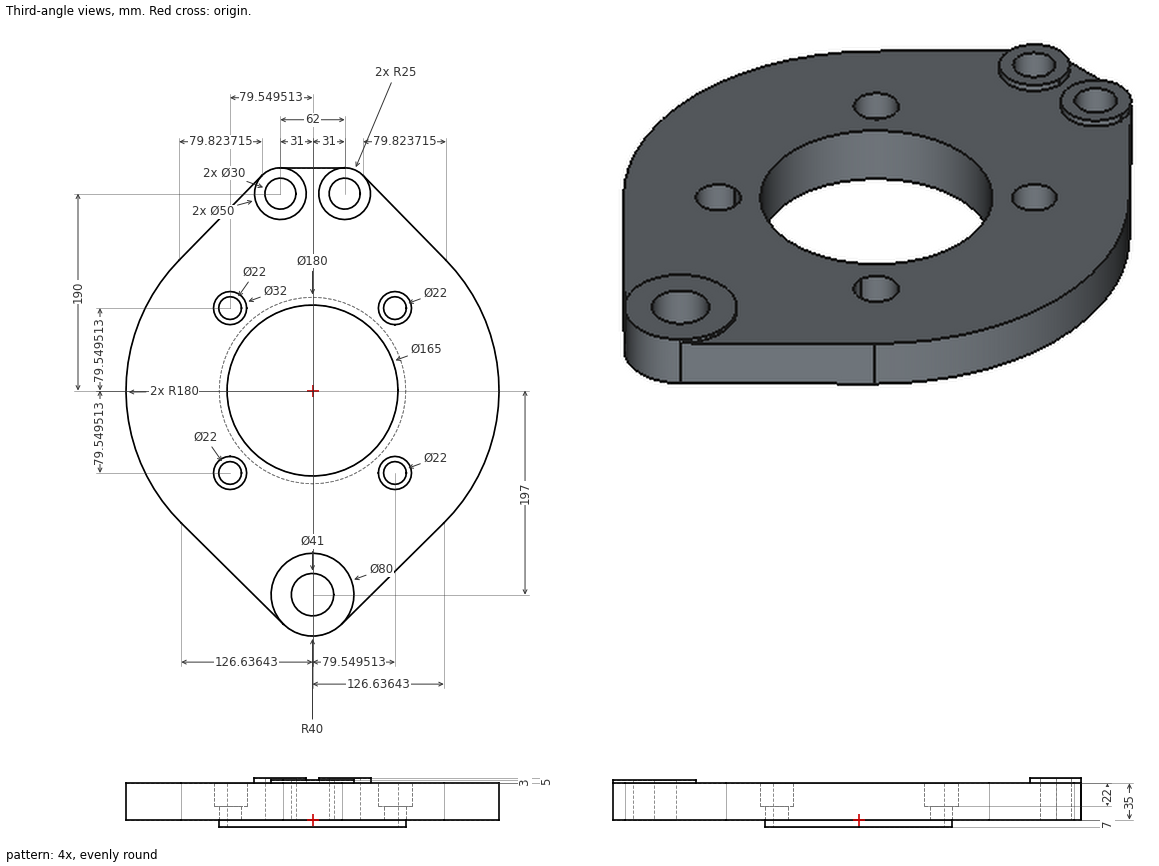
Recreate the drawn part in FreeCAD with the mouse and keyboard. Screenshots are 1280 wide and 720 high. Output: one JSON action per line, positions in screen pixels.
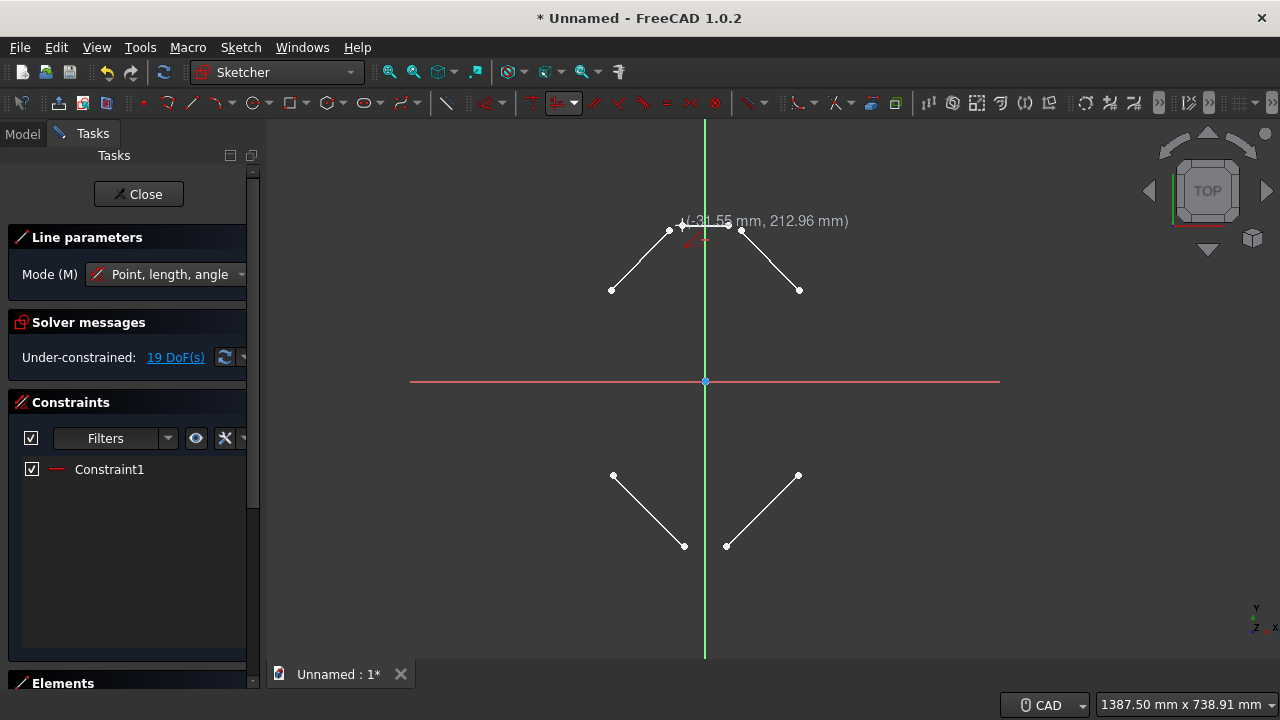
{"action": "key", "text": "g 3 a"}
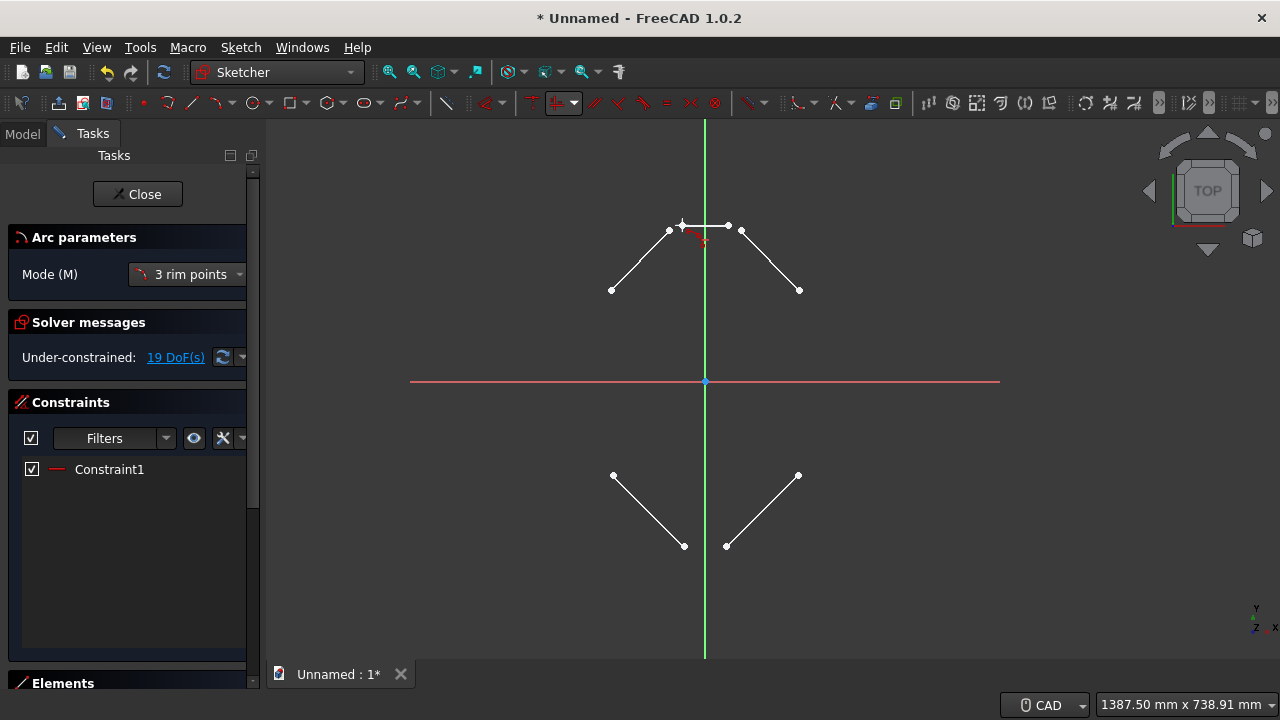
{"action": "left_click", "coordinate": [611, 291]}
{"action": "left_click", "coordinate": [613, 476]}
{"action": "left_click", "coordinate": [575, 362]}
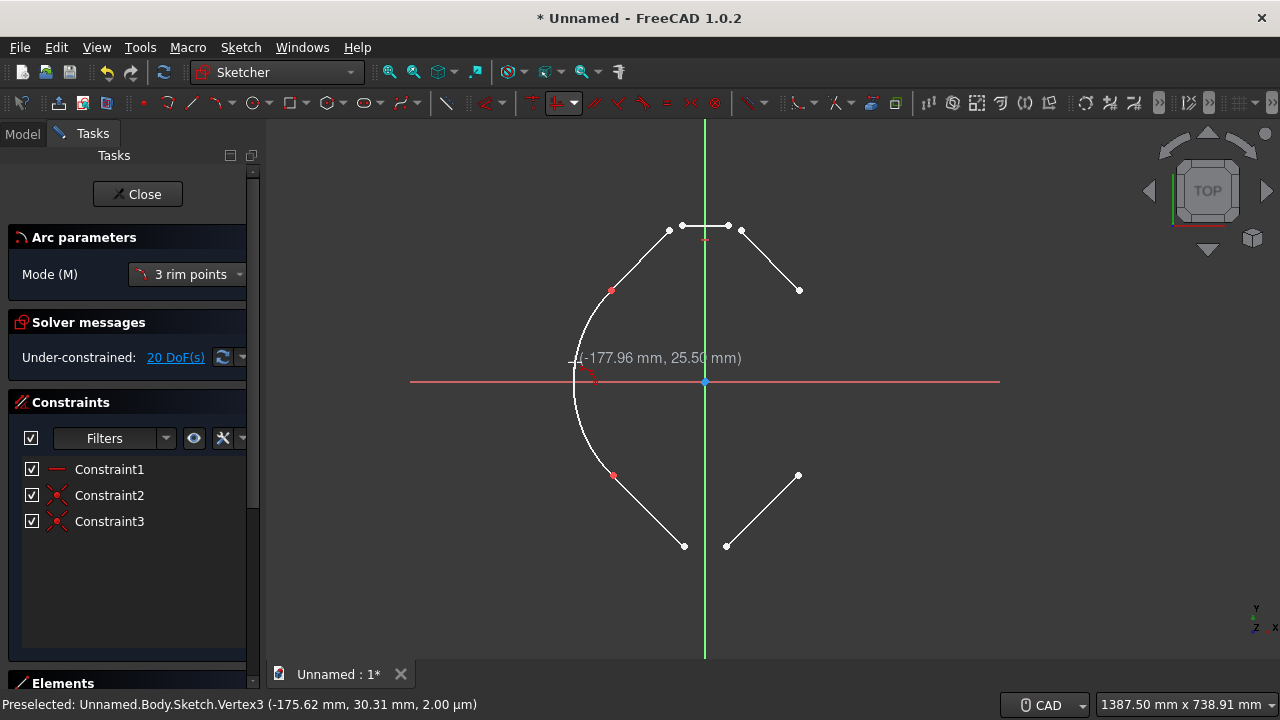
{"action": "left_click", "coordinate": [684, 547]}
{"action": "left_click", "coordinate": [726, 547]}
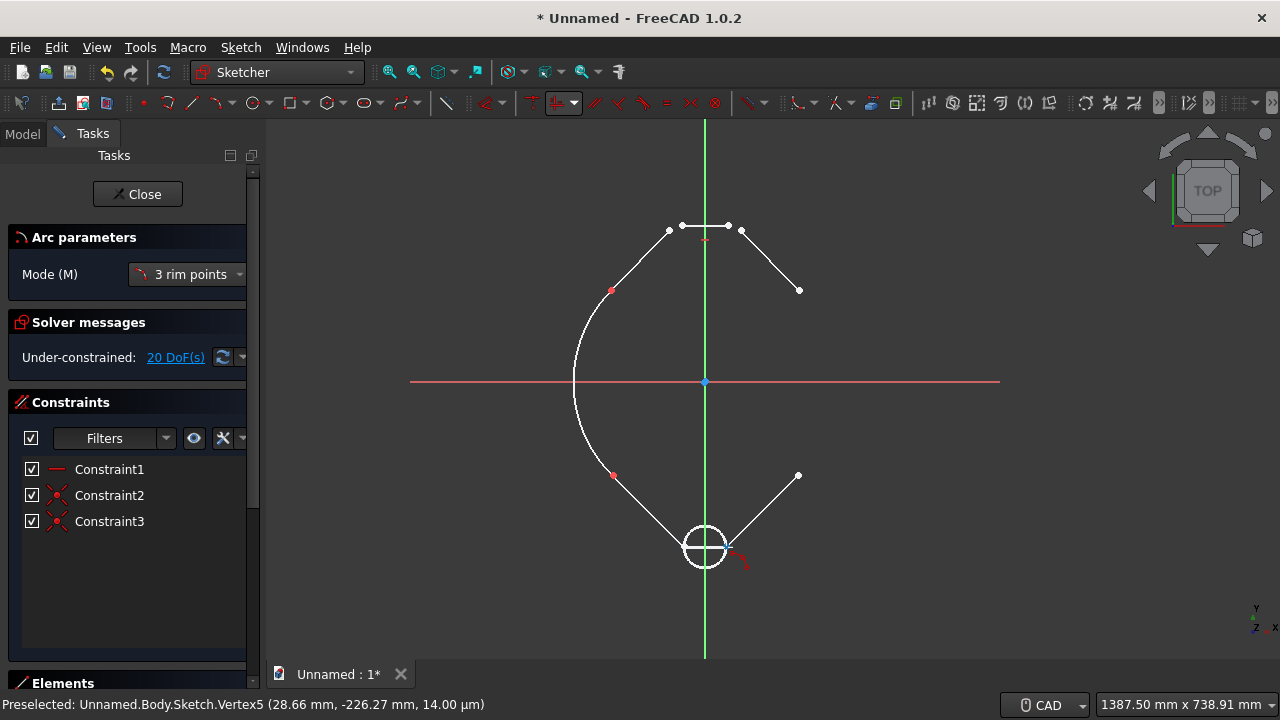
{"action": "scroll", "coordinate": [696, 553], "scroll_direction": "up", "scroll_amount": 5}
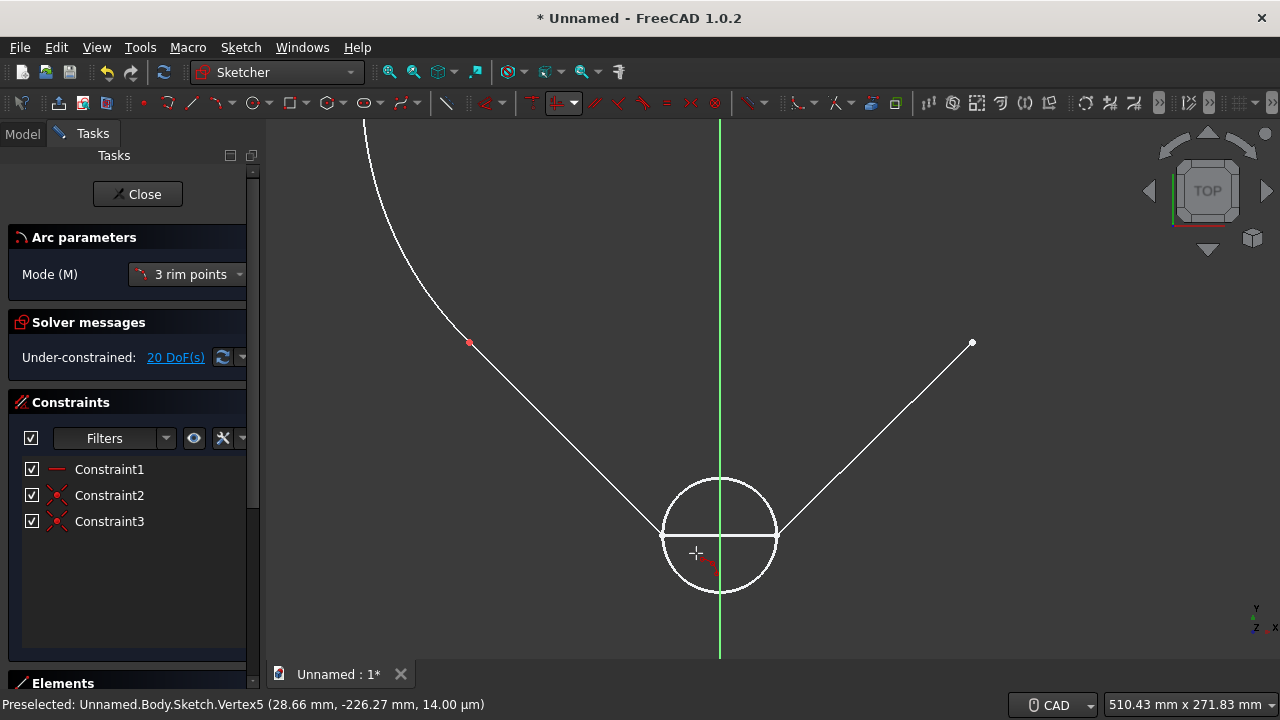
{"action": "left_click", "coordinate": [695, 553]}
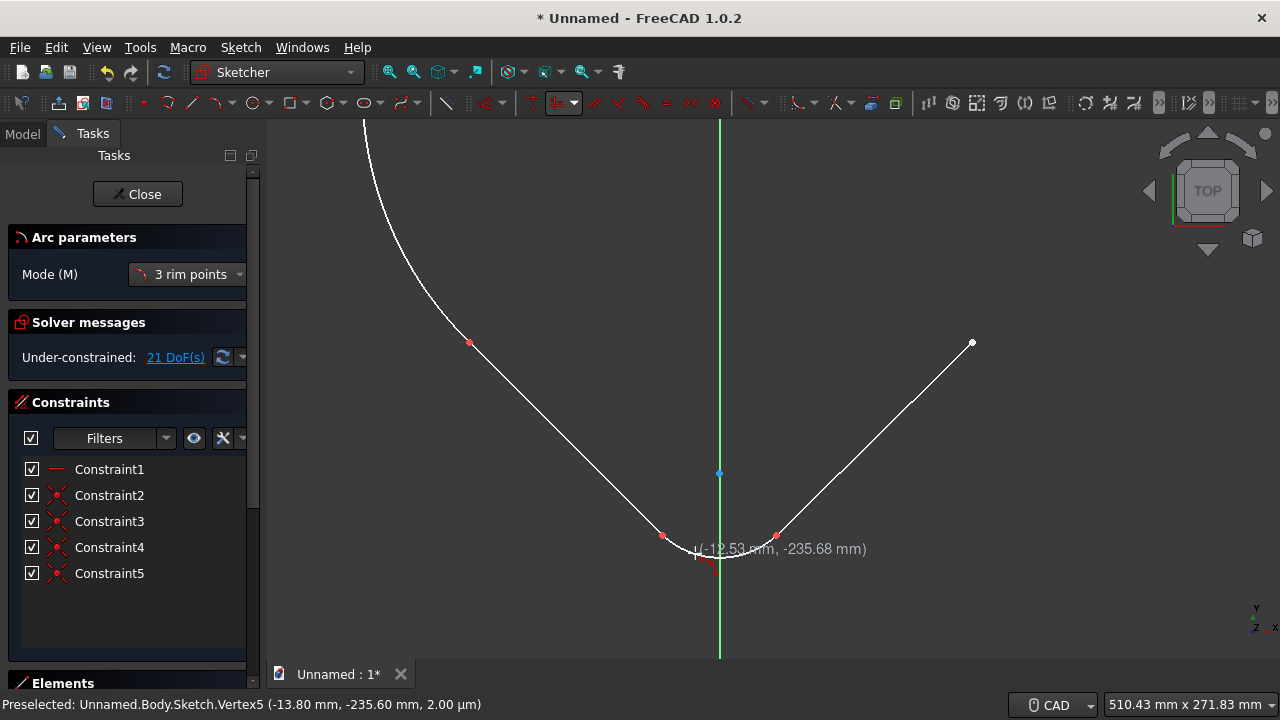
{"action": "left_click", "coordinate": [973, 342]}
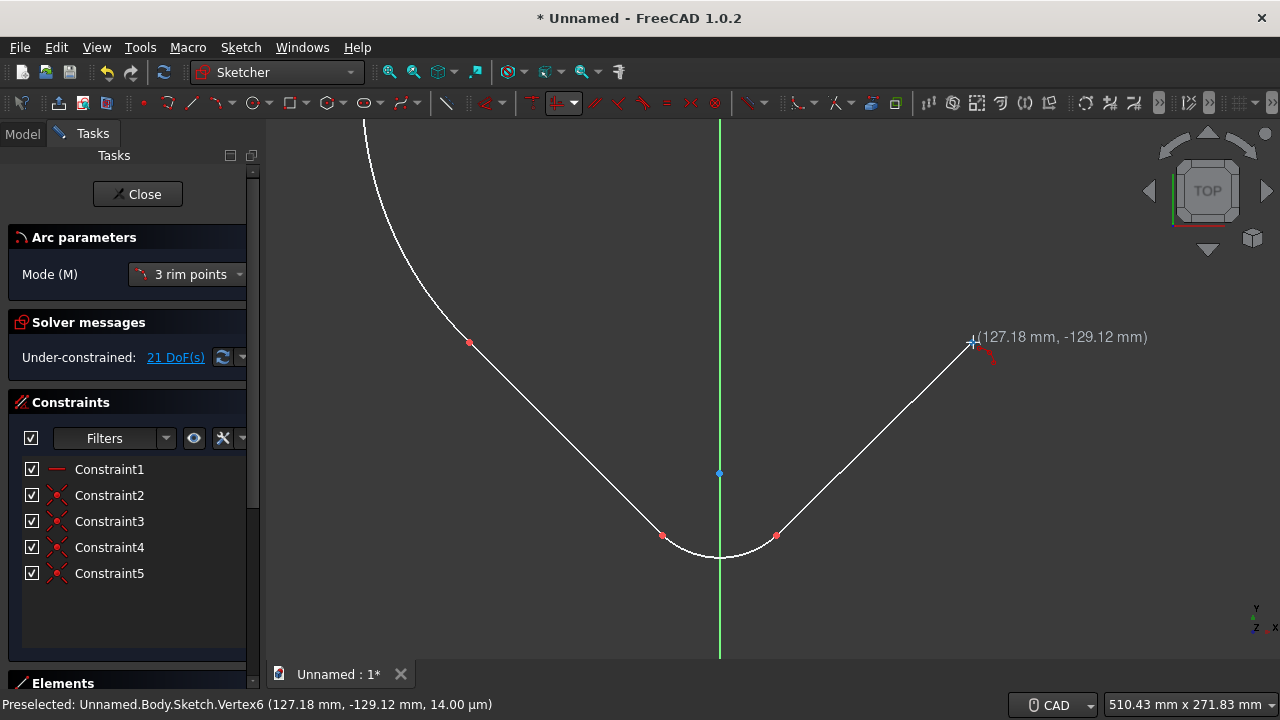
{"action": "scroll", "coordinate": [696, 553], "scroll_direction": "down", "scroll_amount": 5}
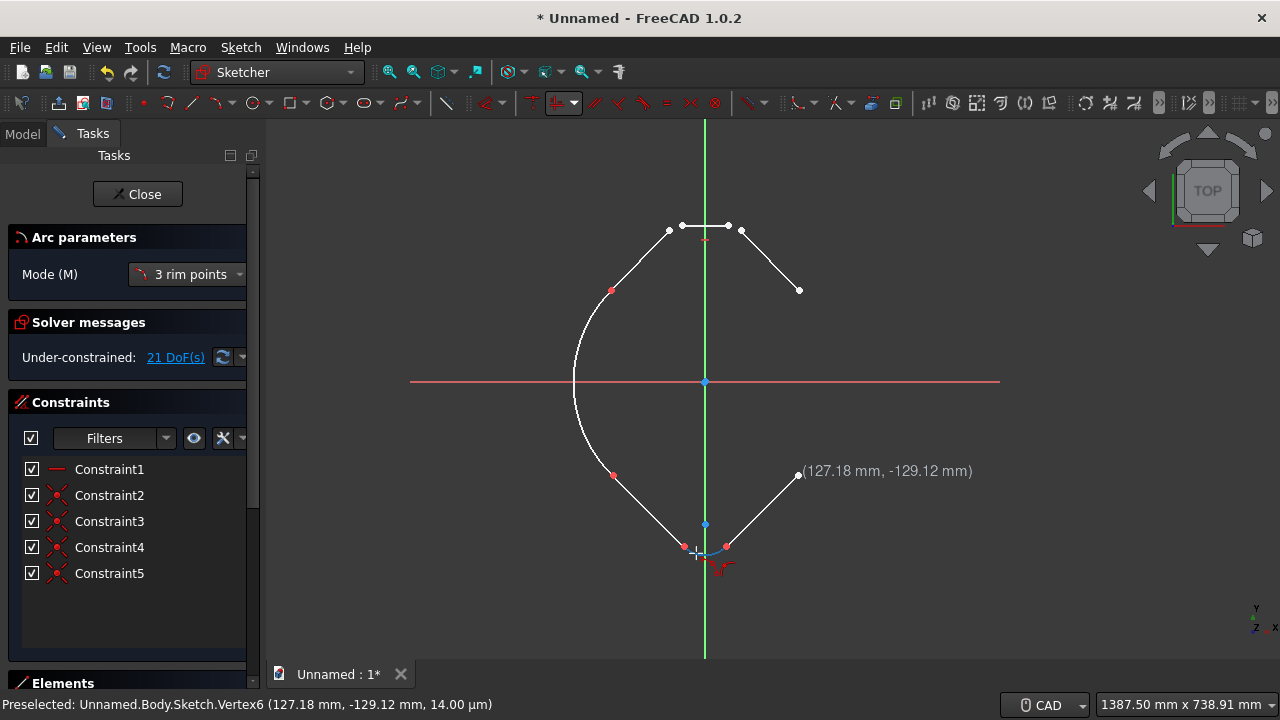
{"action": "left_click", "coordinate": [799, 291]}
{"action": "left_click", "coordinate": [835, 403]}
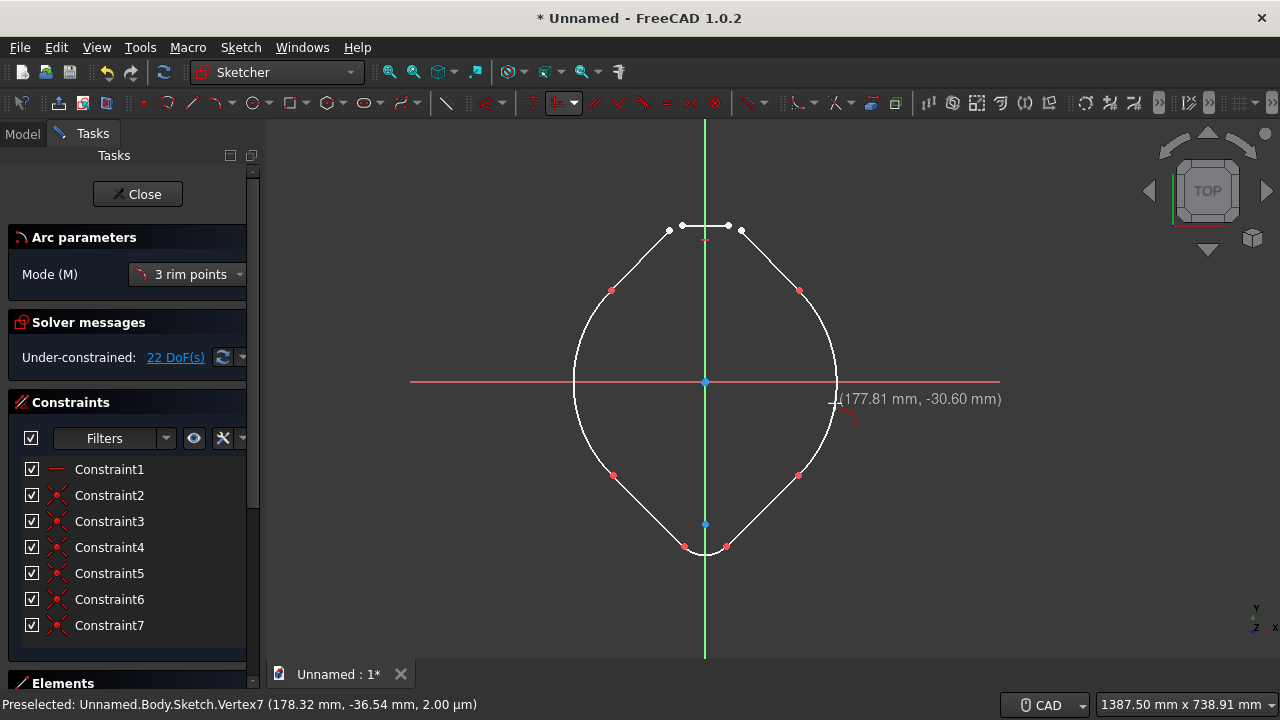
{"action": "left_click", "coordinate": [741, 231]}
{"action": "left_click", "coordinate": [728, 226]}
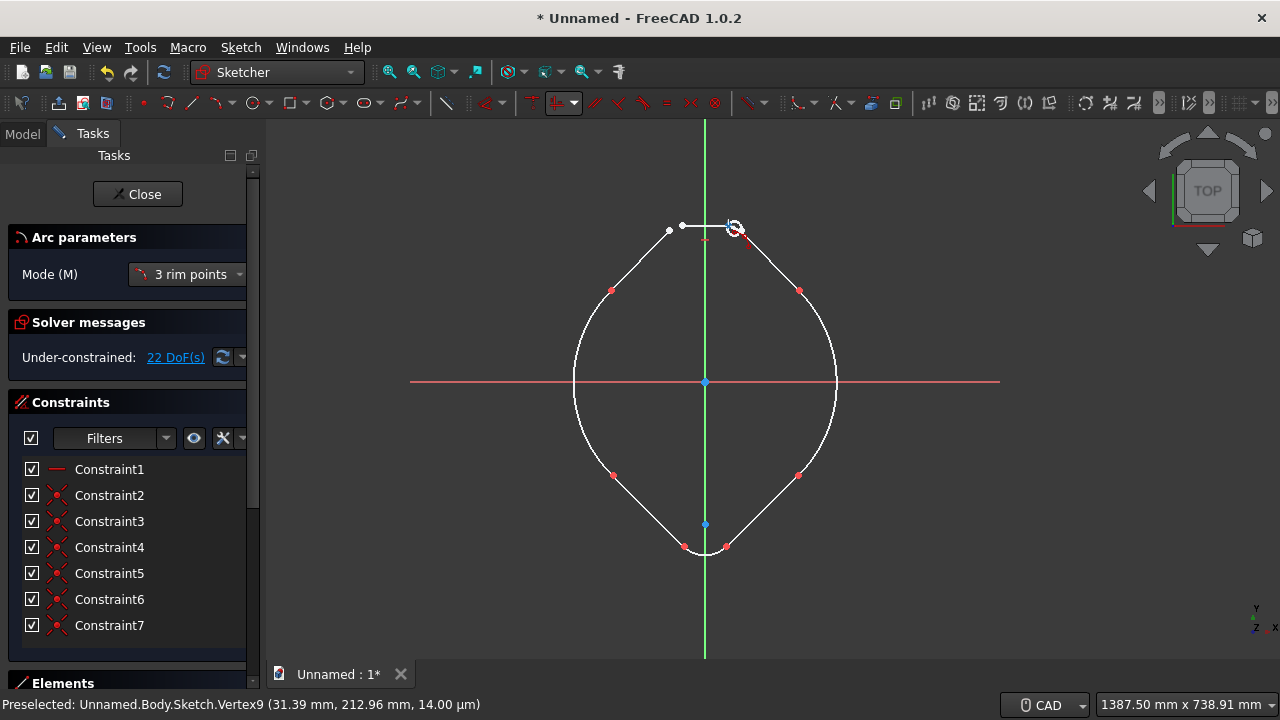
{"action": "scroll", "coordinate": [735, 226], "scroll_direction": "up", "scroll_amount": 13}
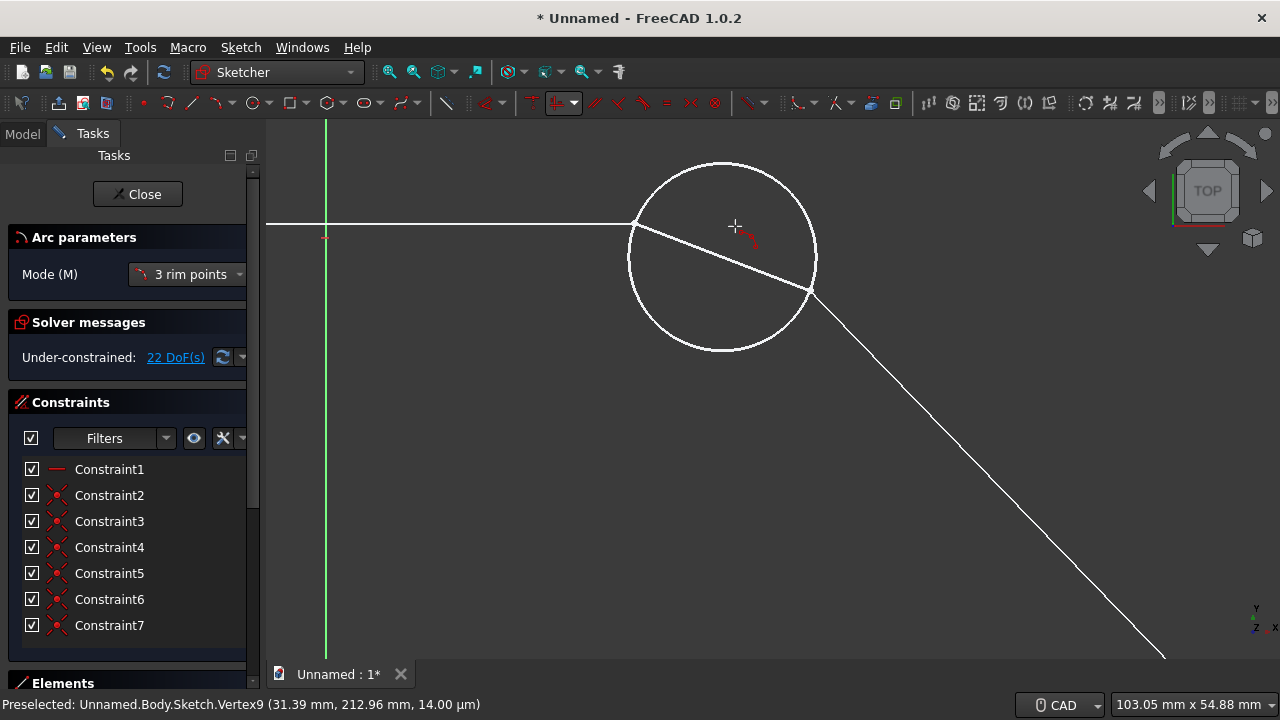
{"action": "left_click", "coordinate": [727, 223]}